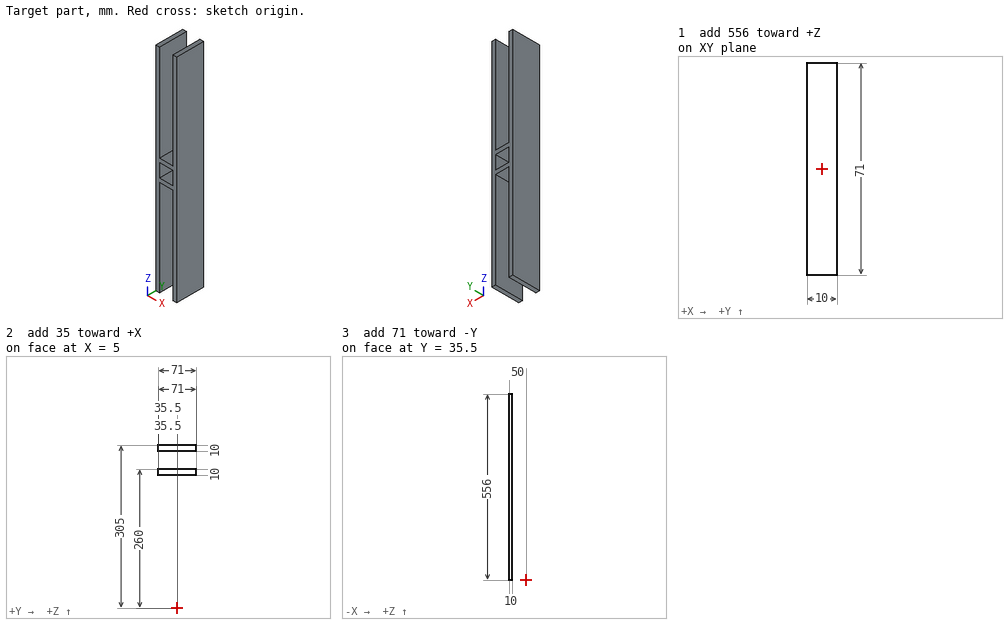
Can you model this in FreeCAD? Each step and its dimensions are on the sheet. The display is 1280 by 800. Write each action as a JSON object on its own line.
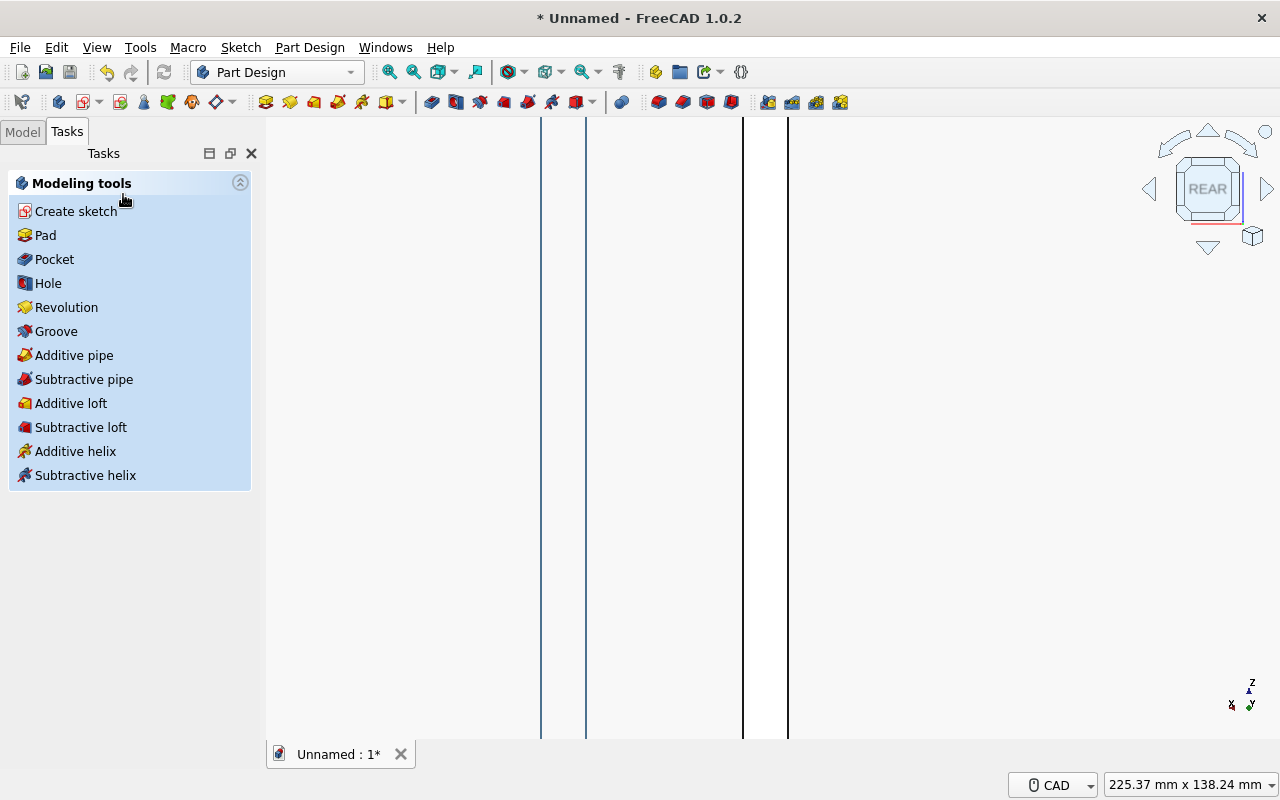
{"action": "left_click", "coordinate": [266, 102]}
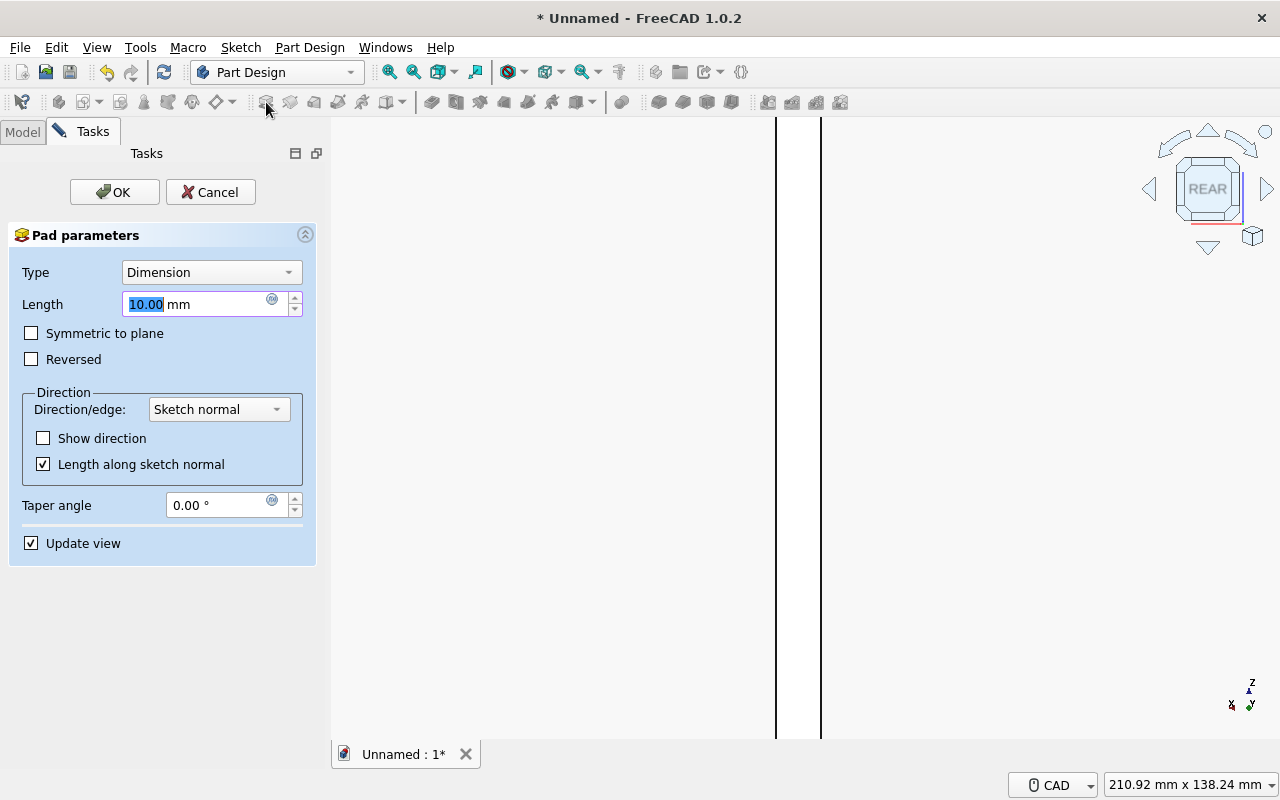
{"action": "type", "text": "71"}
{"action": "key", "text": "Tab"}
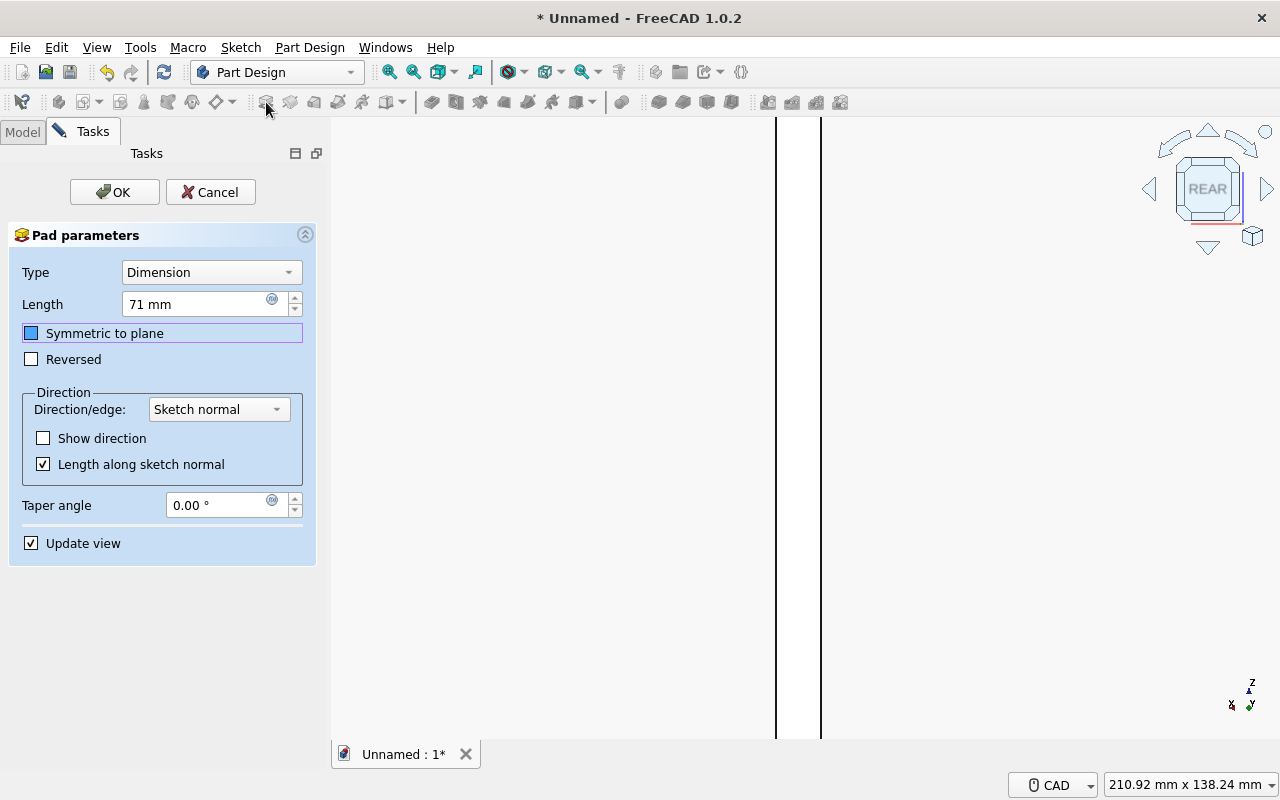
{"action": "left_click", "coordinate": [30, 359]}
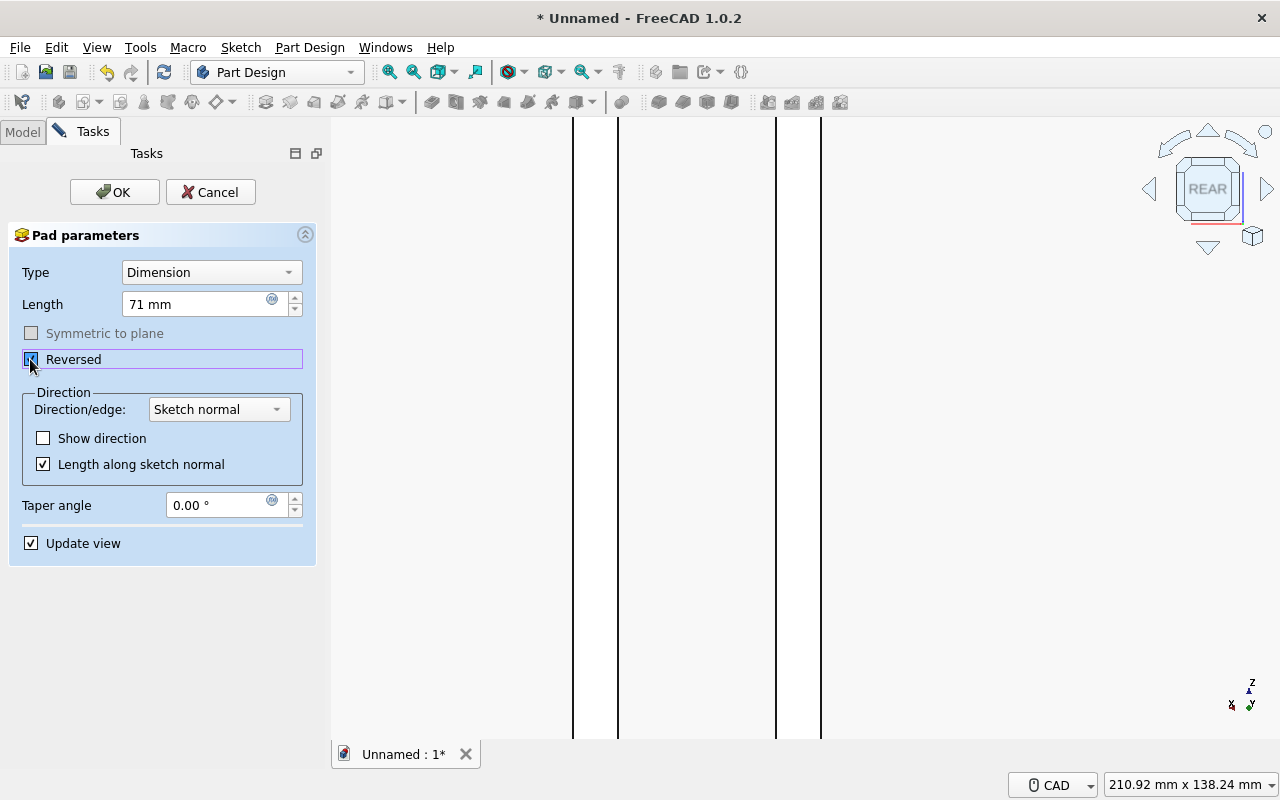
{"action": "left_click", "coordinate": [115, 192]}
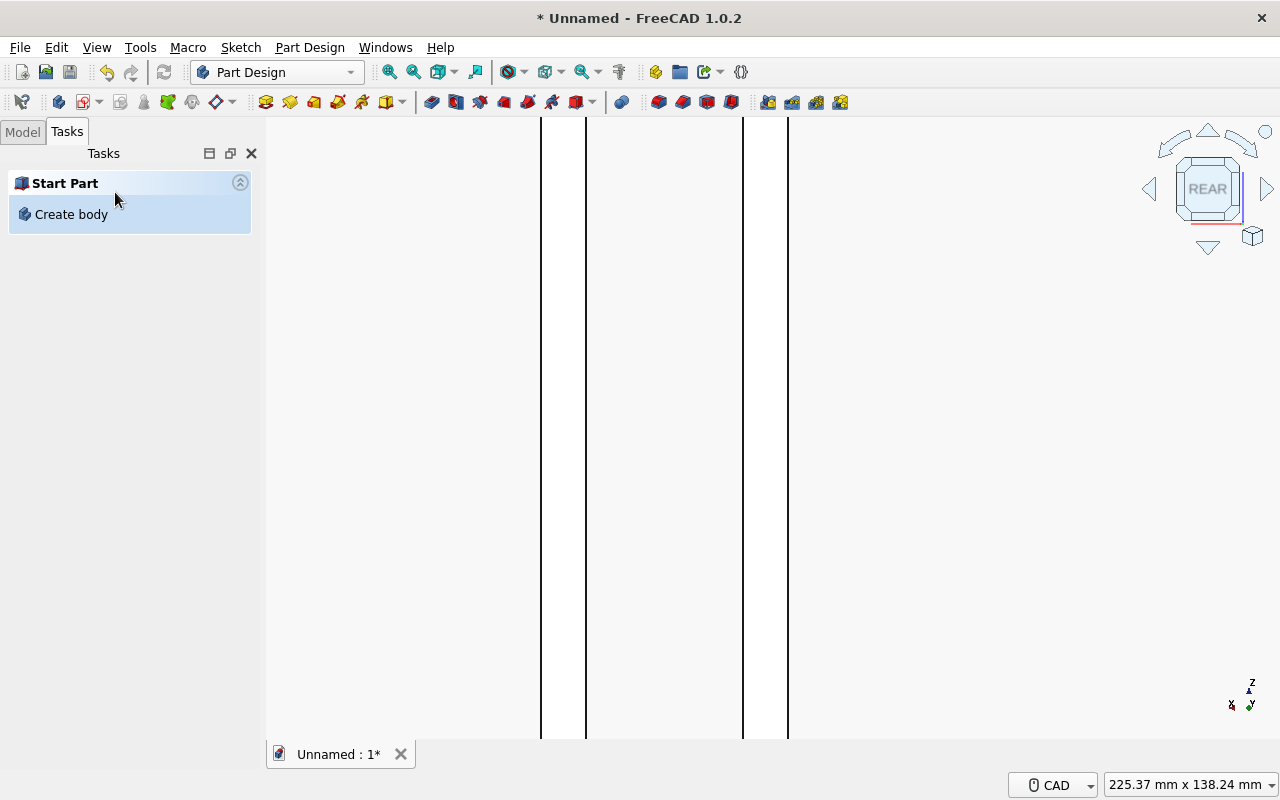
{"action": "key", "text": "0"}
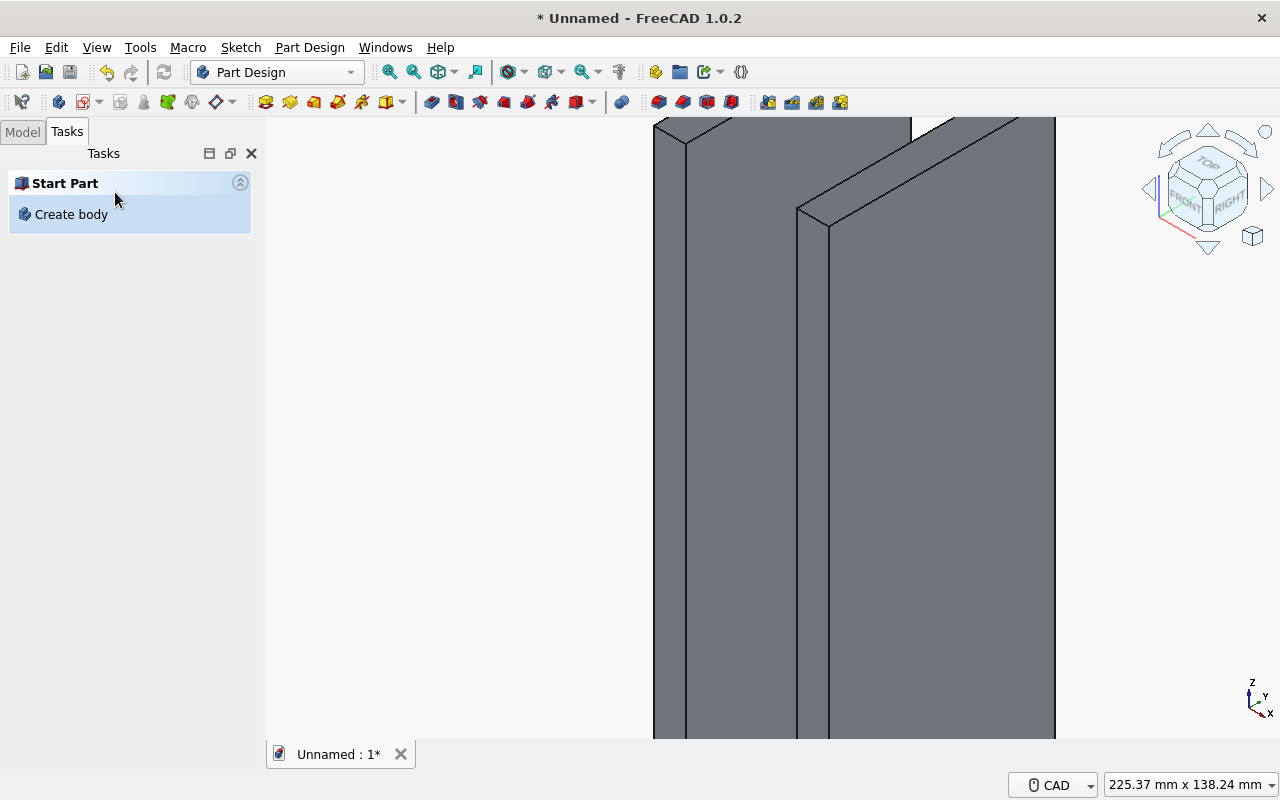
{"action": "key", "text": "v f"}